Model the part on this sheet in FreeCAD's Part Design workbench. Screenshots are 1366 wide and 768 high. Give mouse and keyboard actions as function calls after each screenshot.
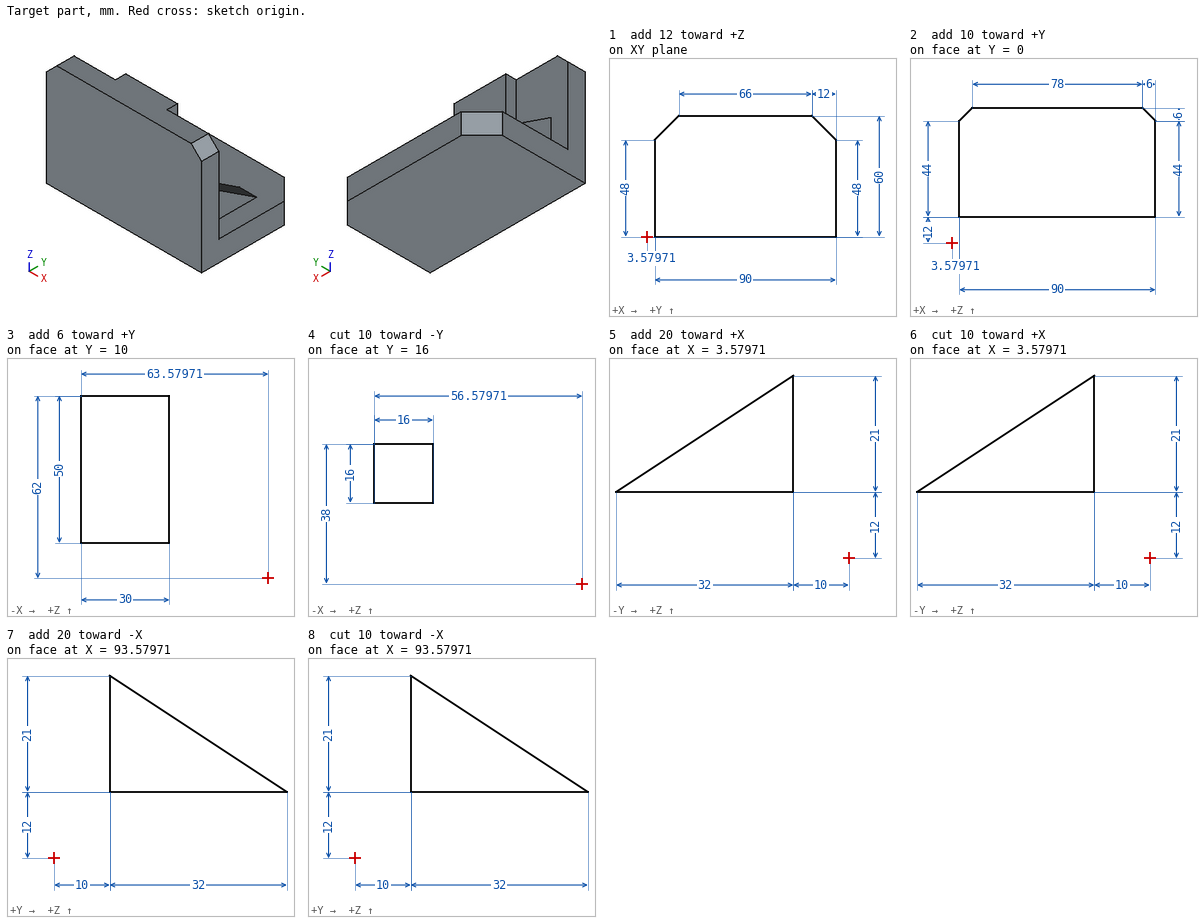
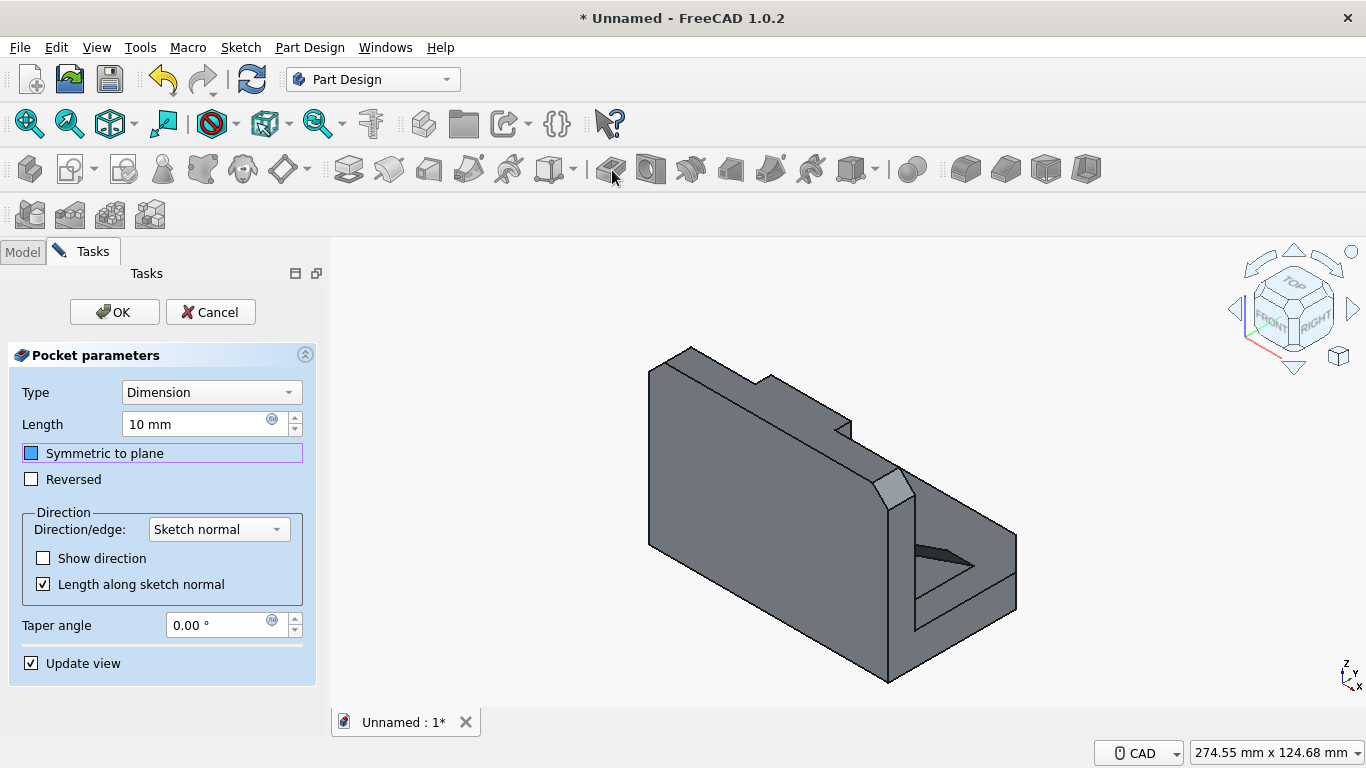
click(115, 312)